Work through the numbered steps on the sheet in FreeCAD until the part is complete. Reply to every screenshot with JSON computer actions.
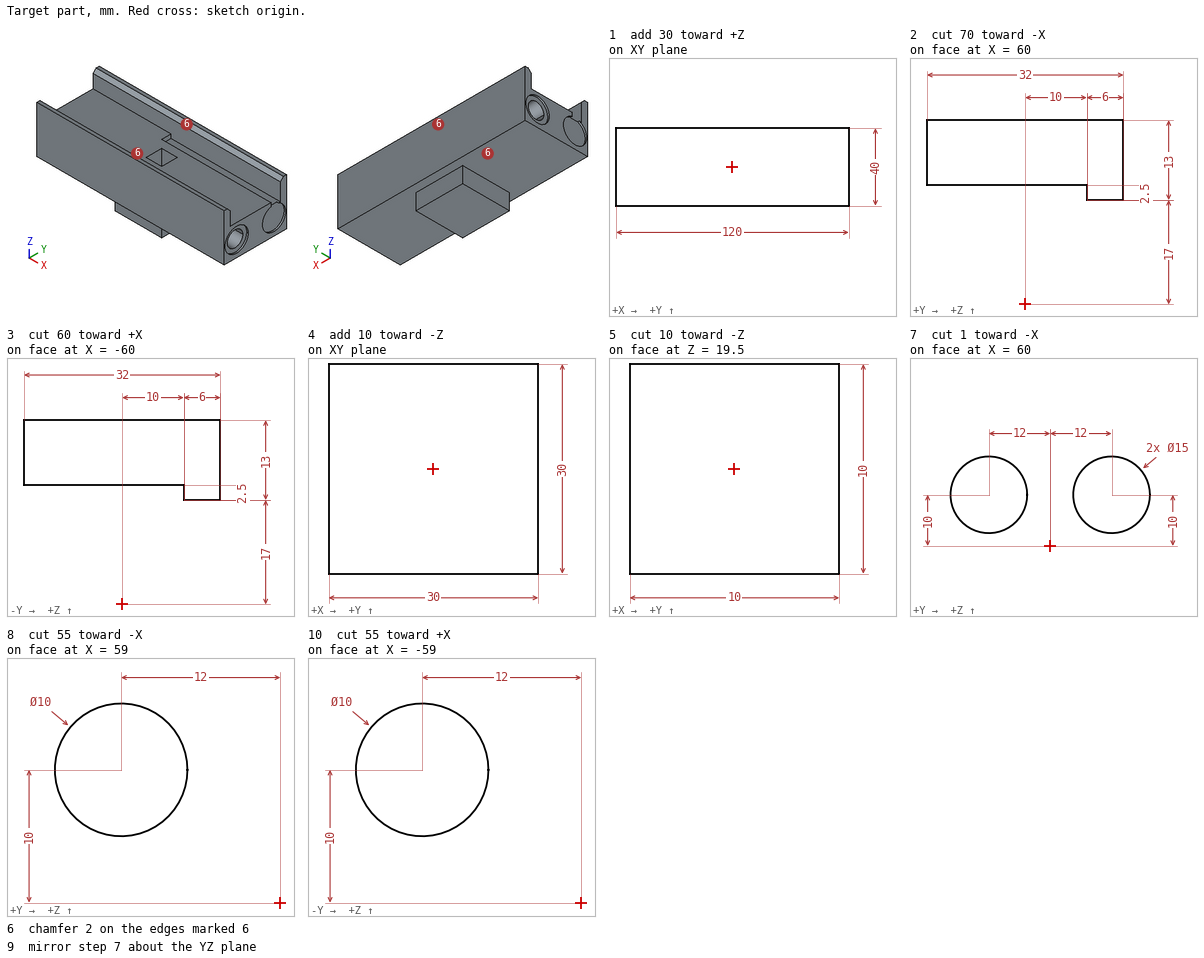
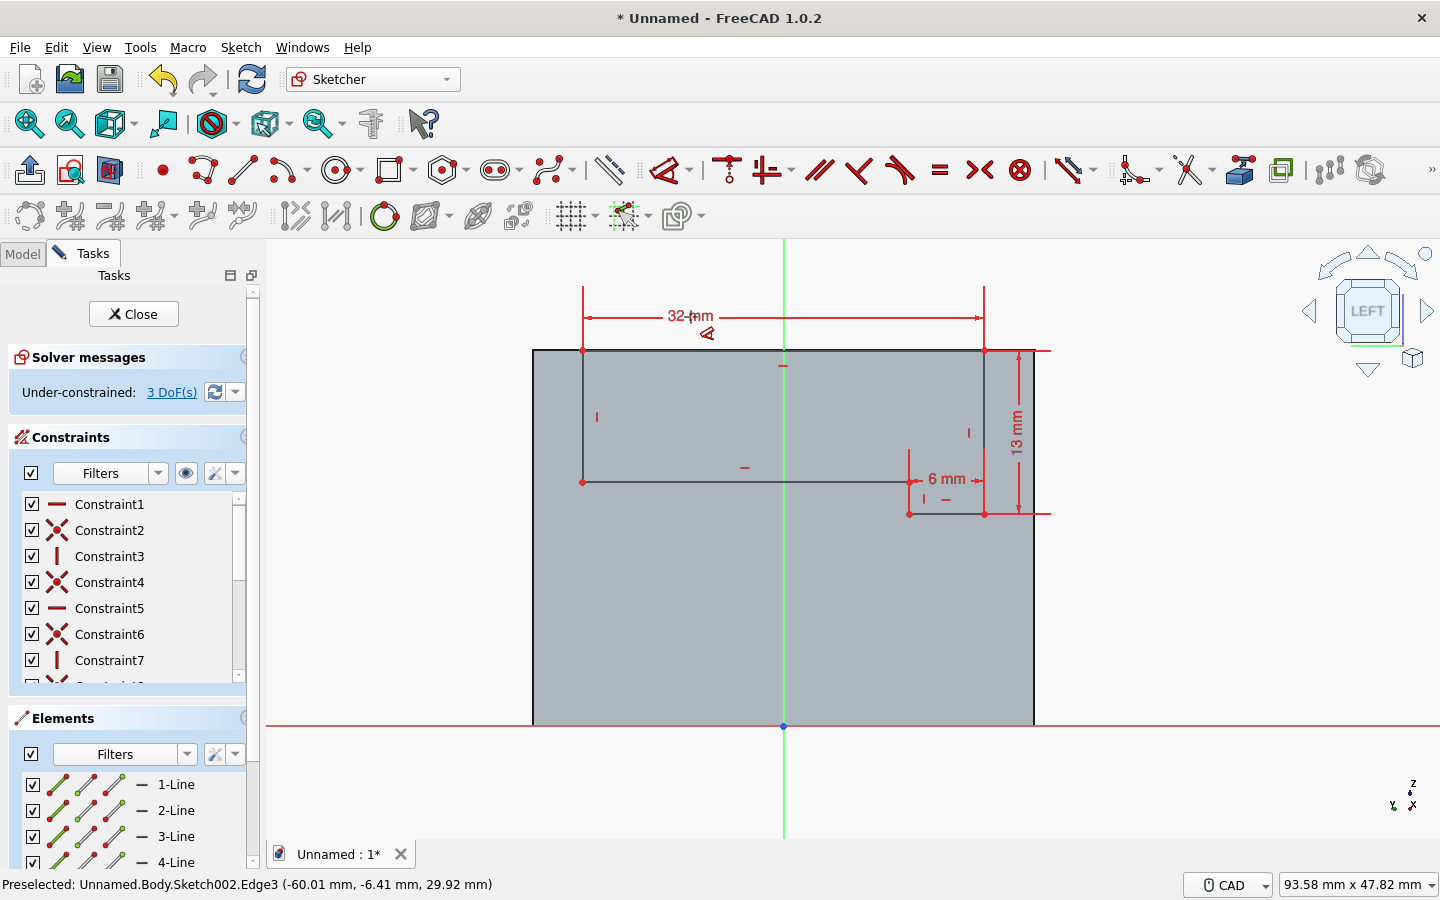
{"action": "scroll", "coordinate": [909, 492], "scroll_direction": "up", "scroll_amount": 2}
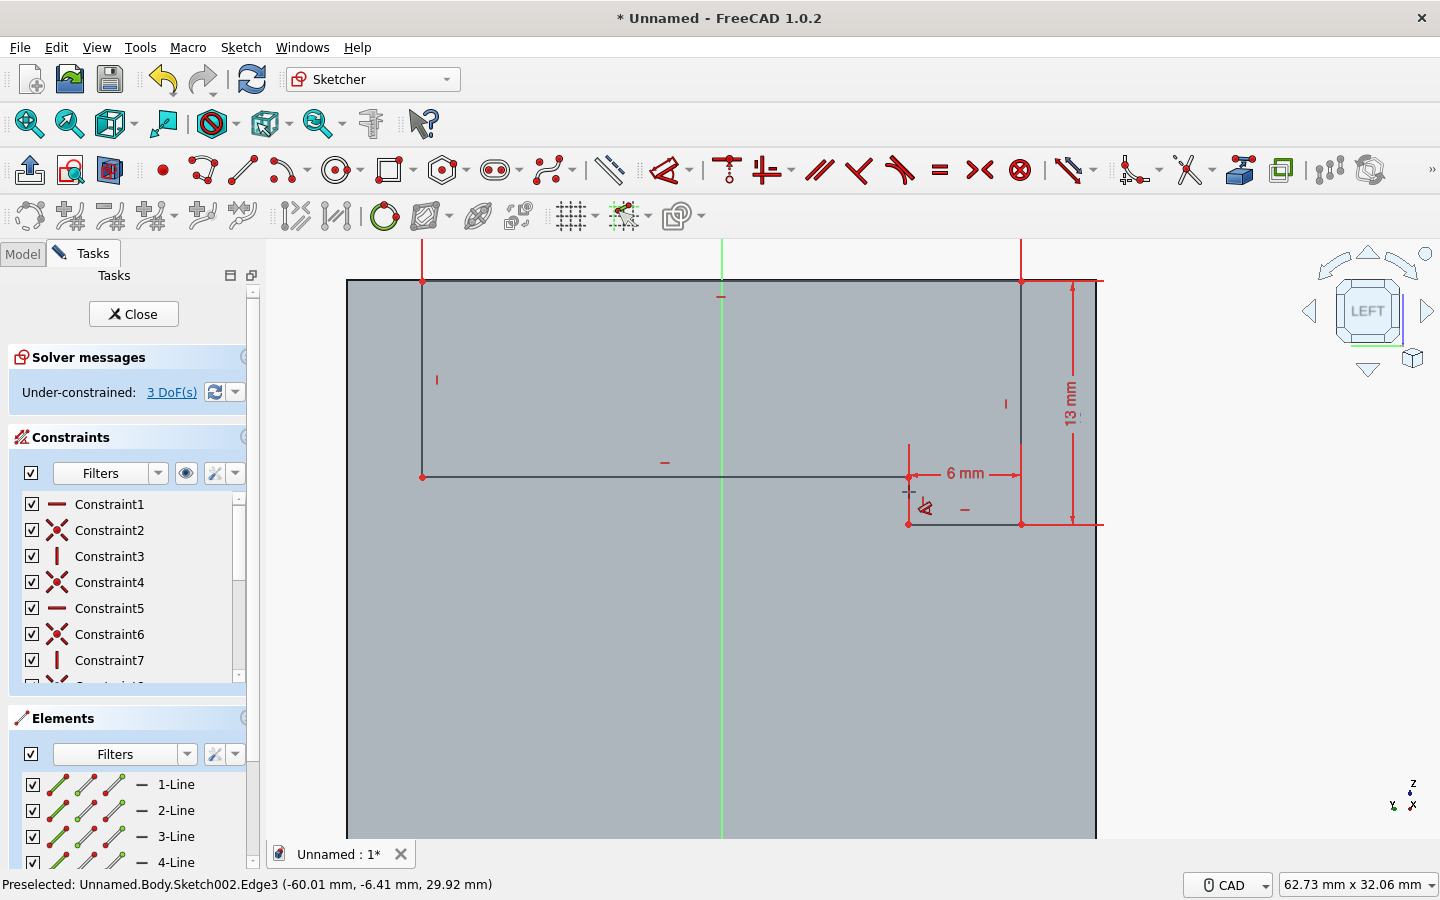
{"action": "left_click", "coordinate": [909, 491]}
{"action": "left_click", "coordinate": [943, 501]}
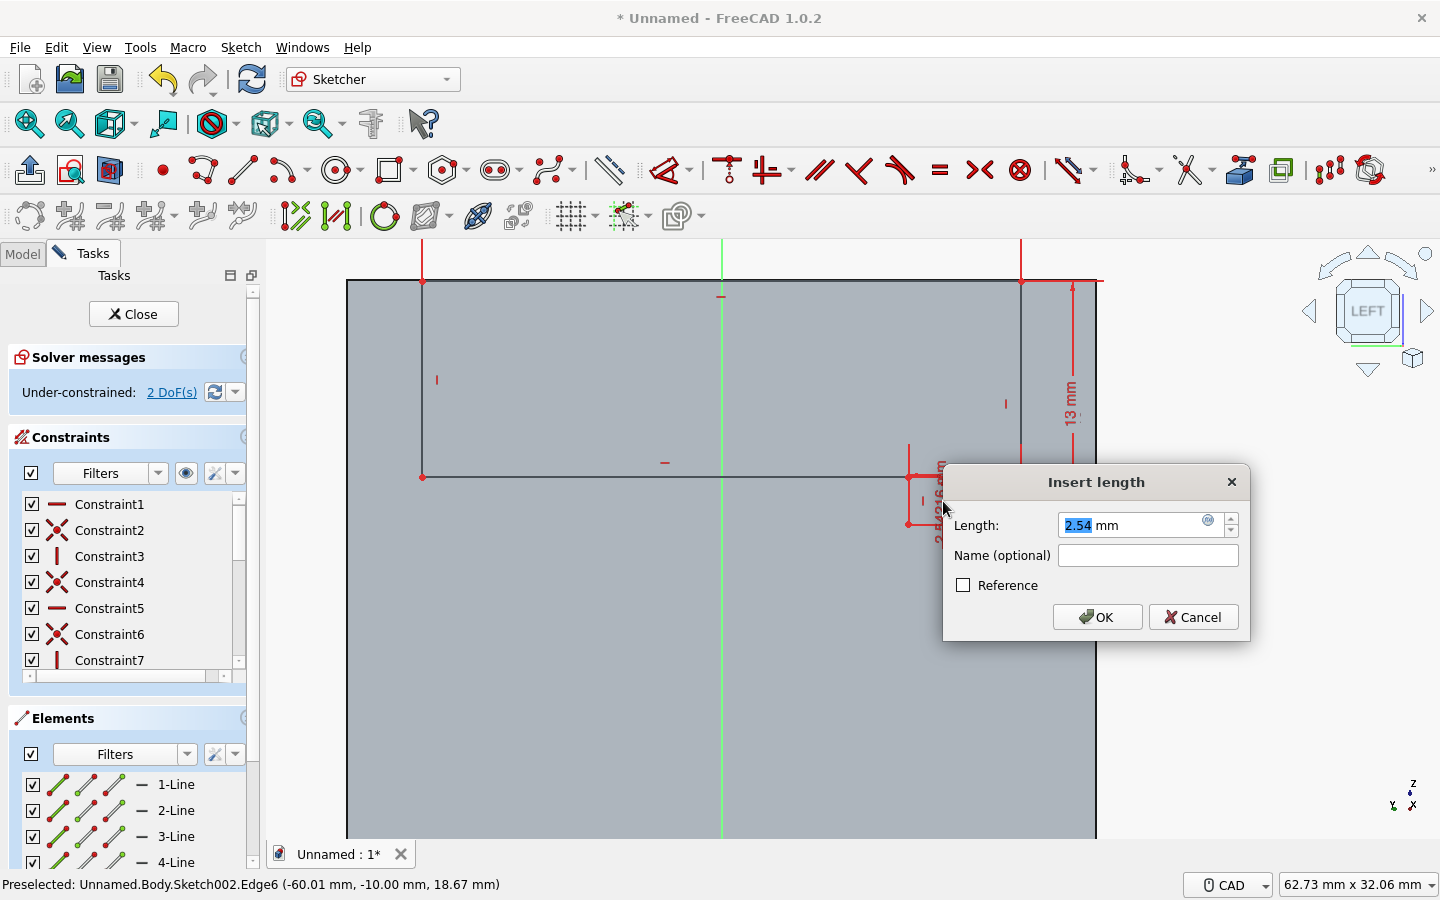
{"action": "type", "text": "2.5"}
{"action": "key", "text": "Return"}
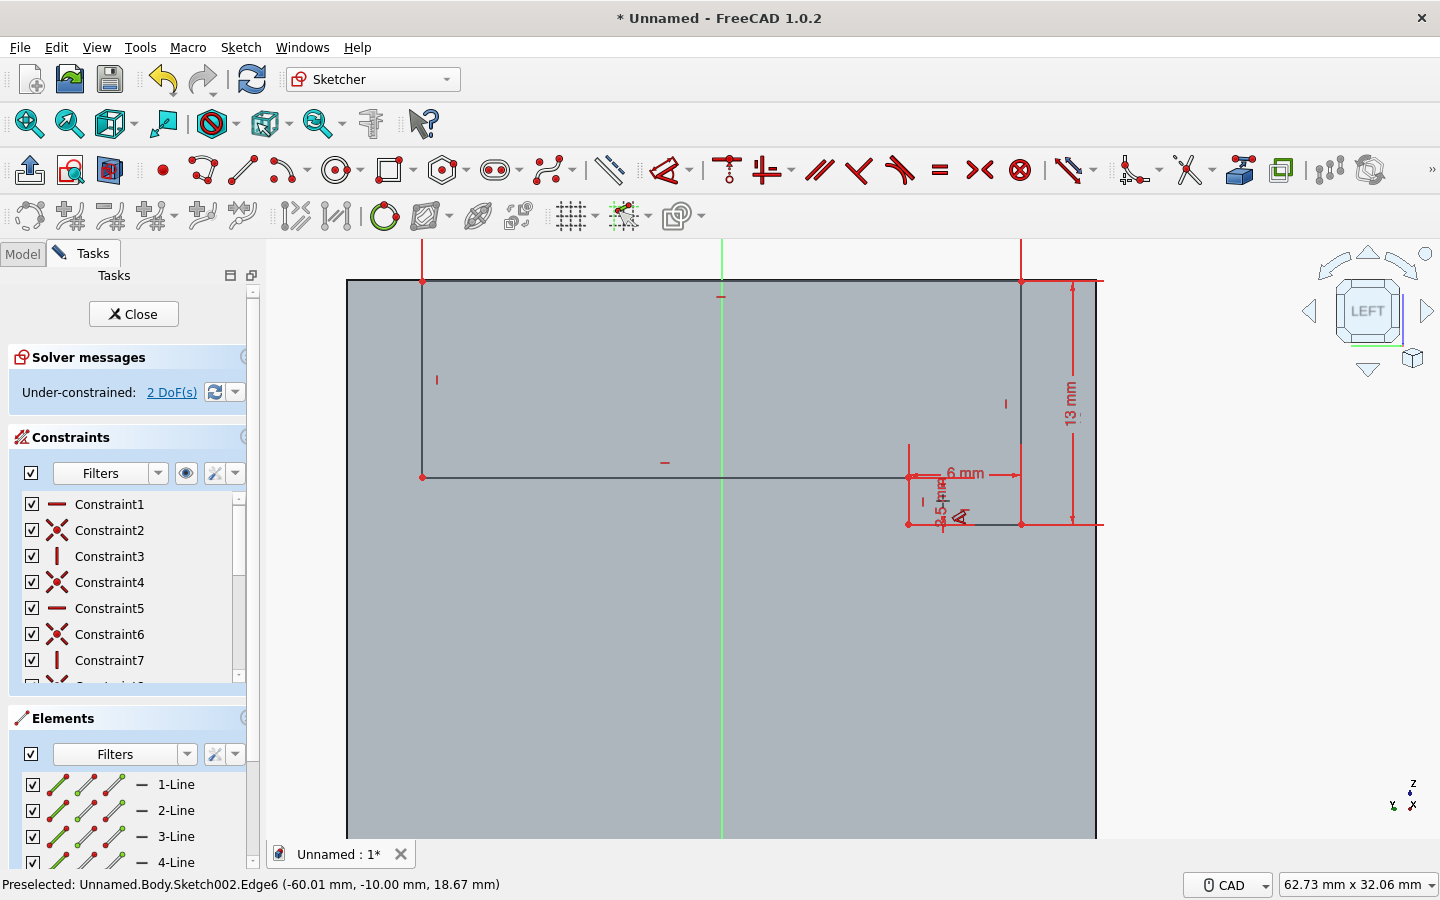
{"action": "left_click", "coordinate": [909, 525]}
{"action": "left_click", "coordinate": [815, 443]}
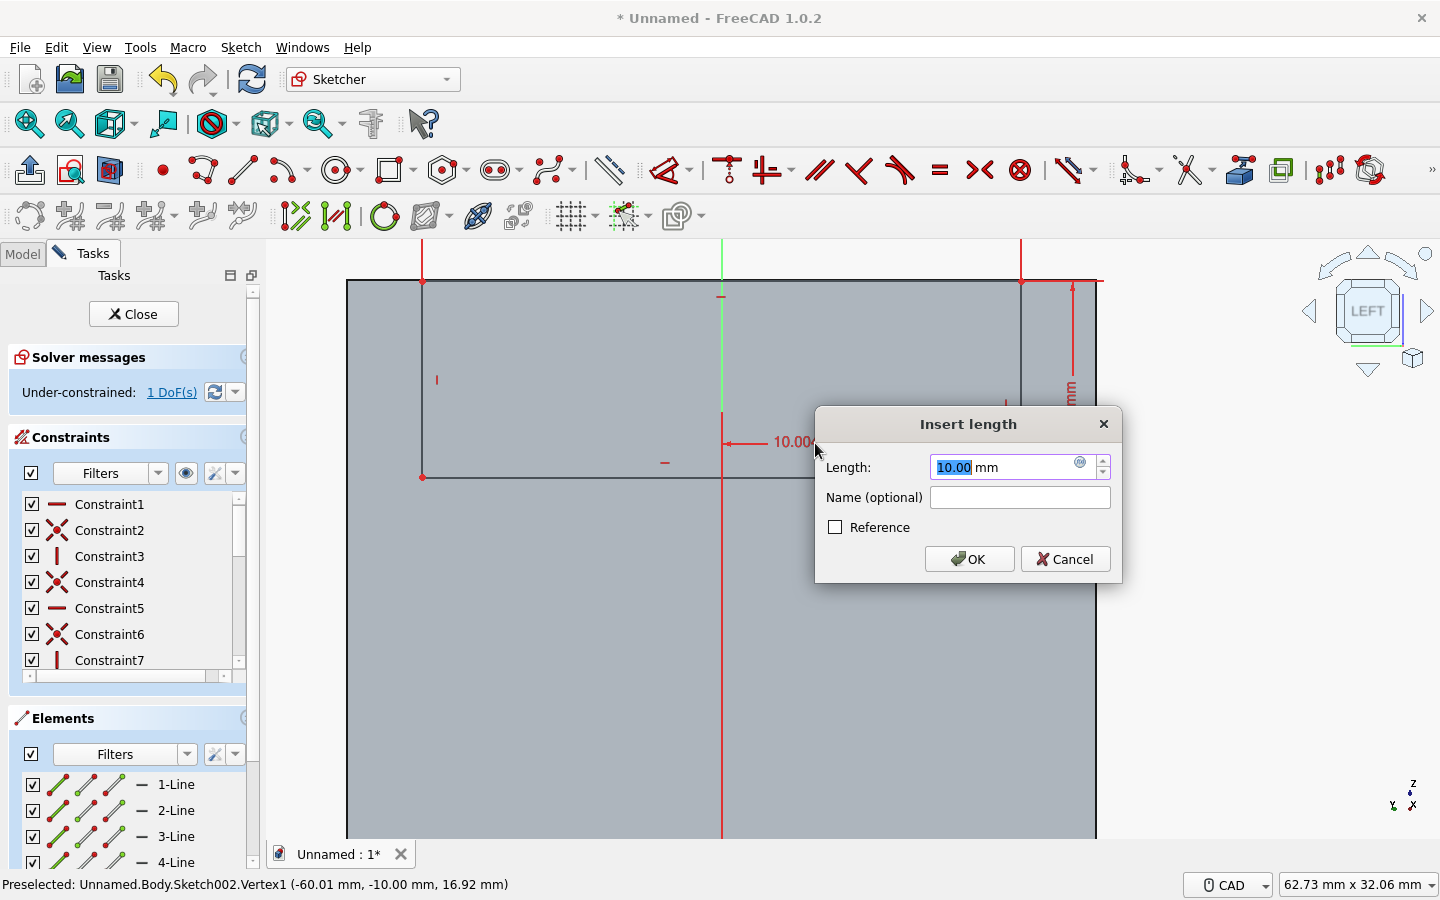
{"action": "type", "text": "10"}
{"action": "key", "text": "Return"}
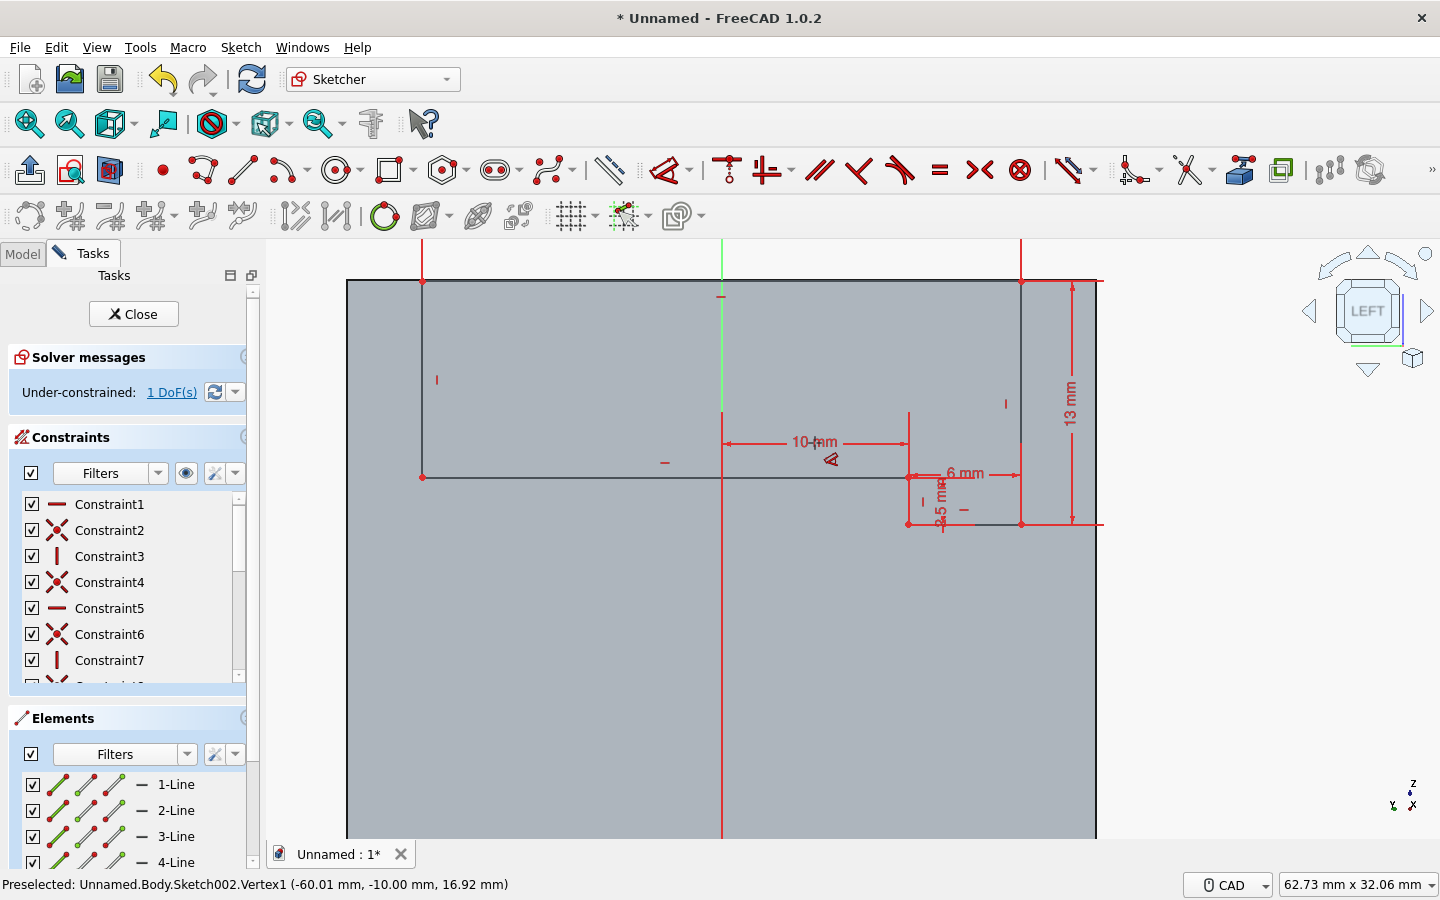
{"action": "left_click", "coordinate": [909, 525]}
{"action": "left_click", "coordinate": [943, 668]}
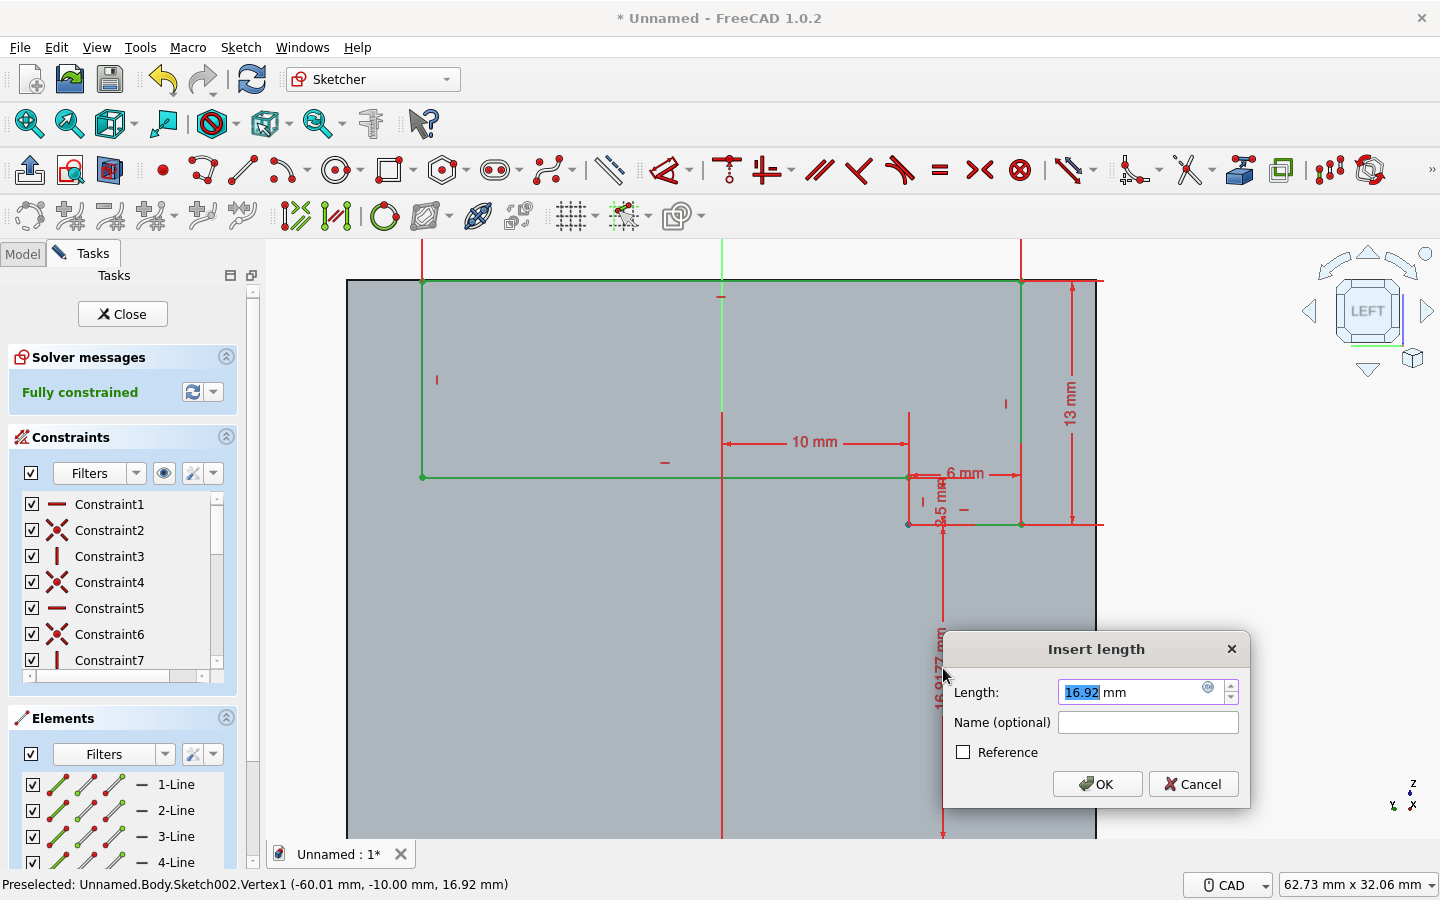
{"action": "type", "text": "17"}
{"action": "key", "text": "Return"}
{"action": "key", "text": "Escape"}